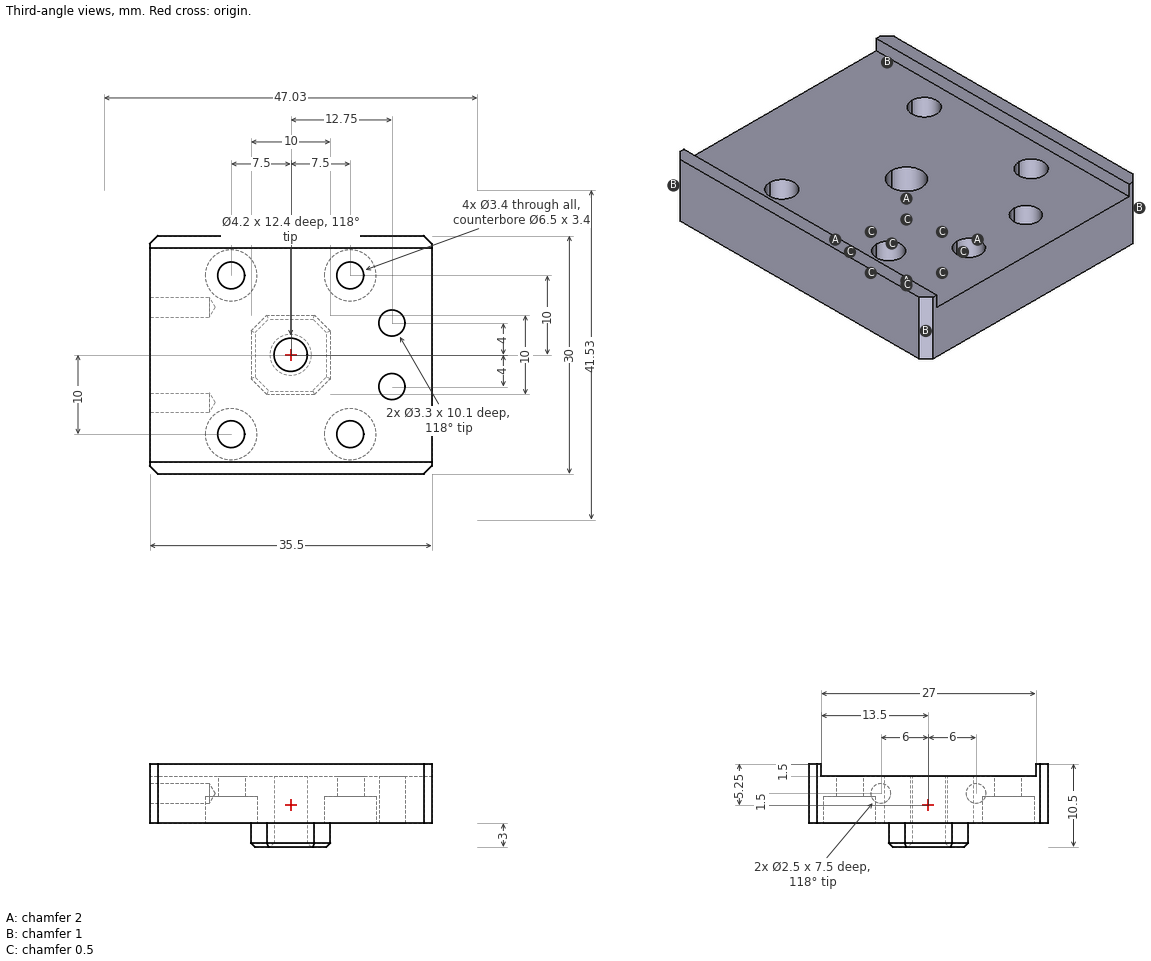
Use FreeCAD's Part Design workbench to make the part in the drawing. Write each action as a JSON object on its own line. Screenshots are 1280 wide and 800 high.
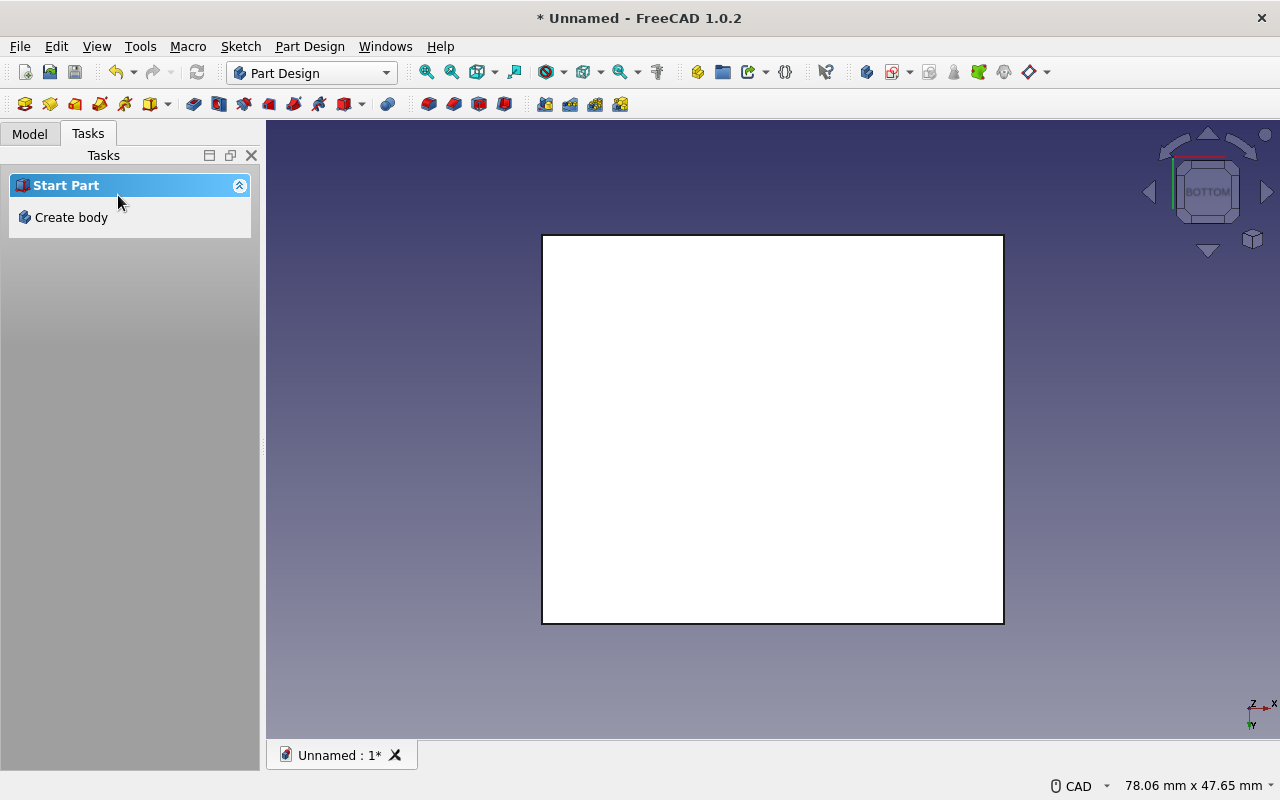
{"action": "left_click", "coordinate": [773, 428]}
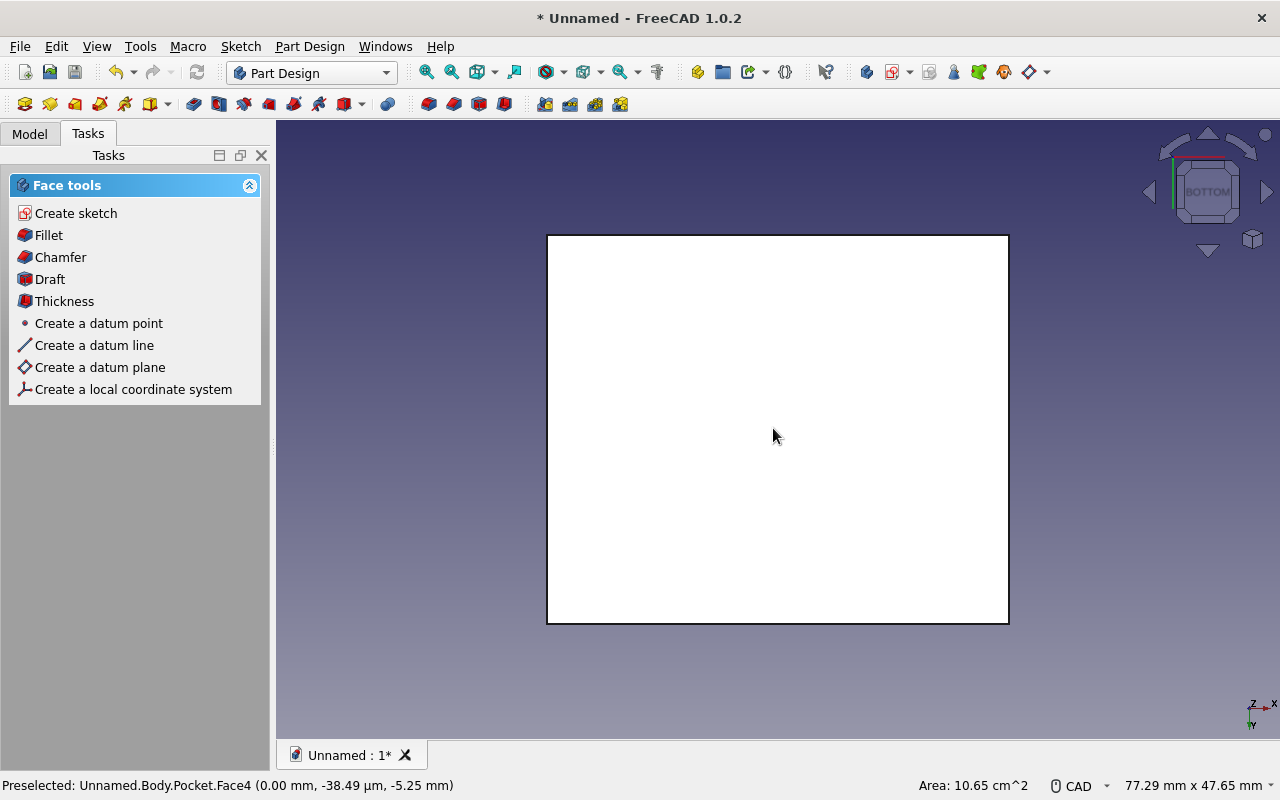
{"action": "left_click", "coordinate": [892, 72]}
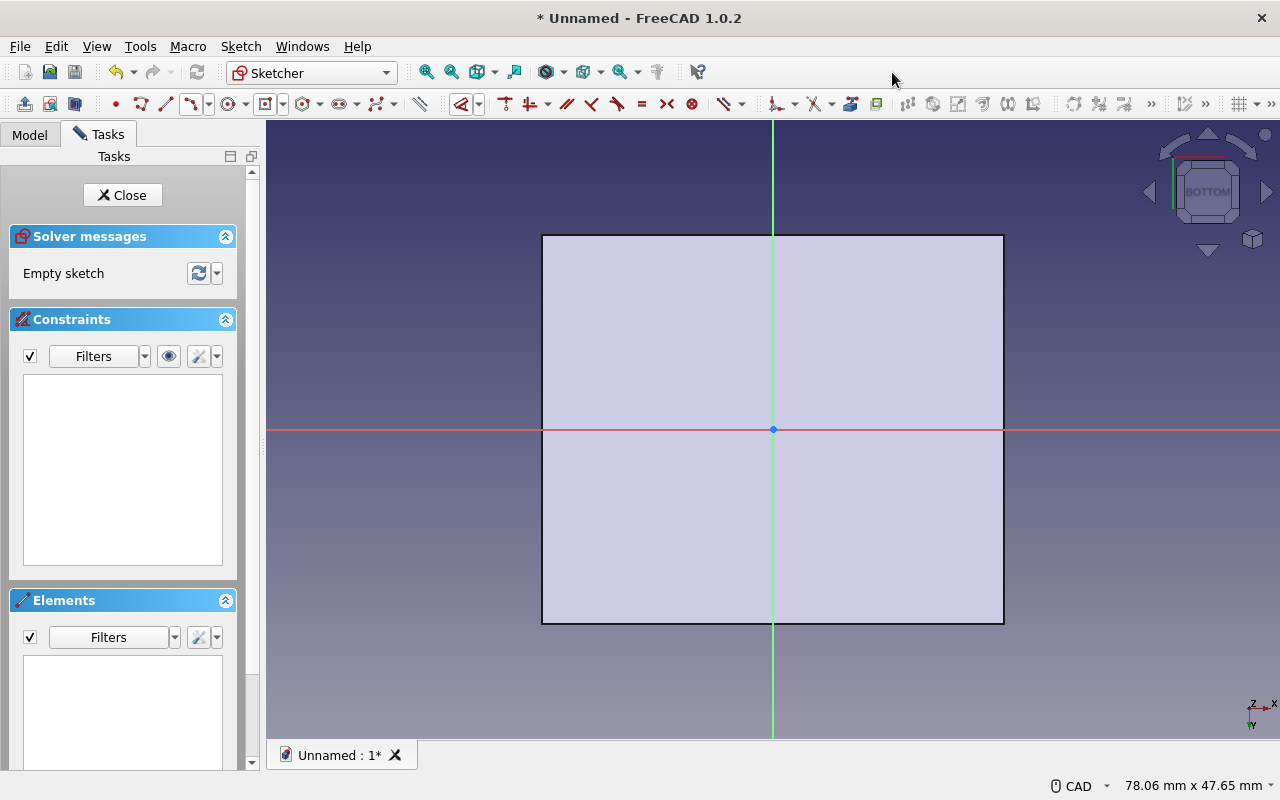
{"action": "scroll", "coordinate": [784, 430], "scroll_direction": "up", "scroll_amount": 10}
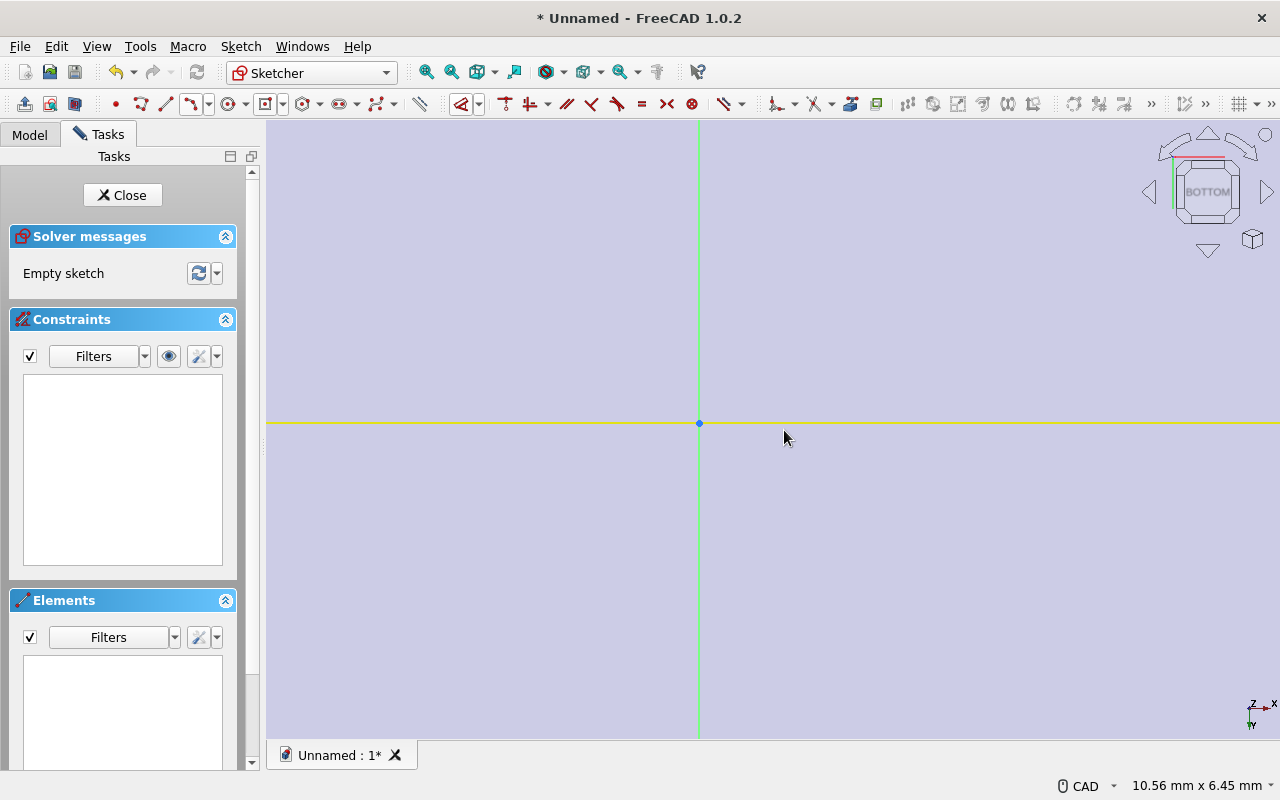
{"action": "key", "text": "g c"}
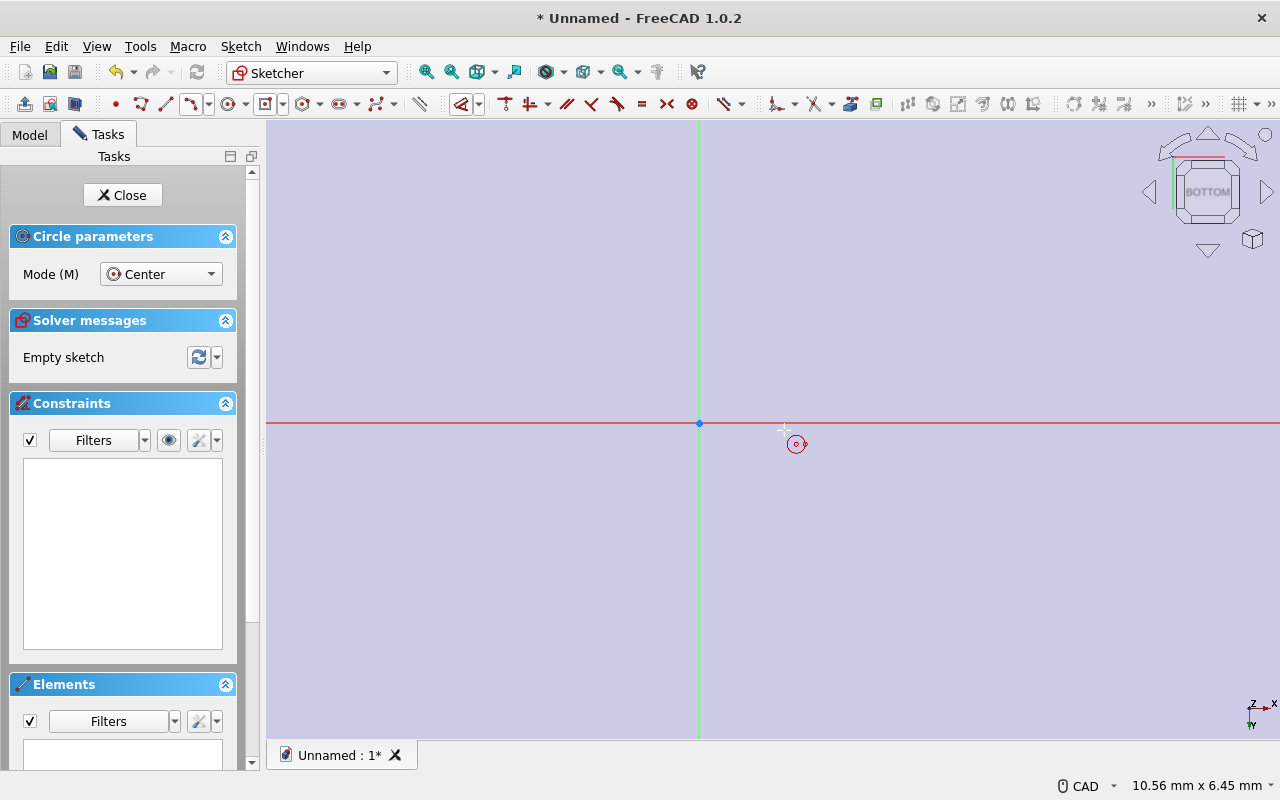
{"action": "left_click", "coordinate": [699, 423]}
{"action": "left_click", "coordinate": [842, 281]}
{"action": "key", "text": "Escape"}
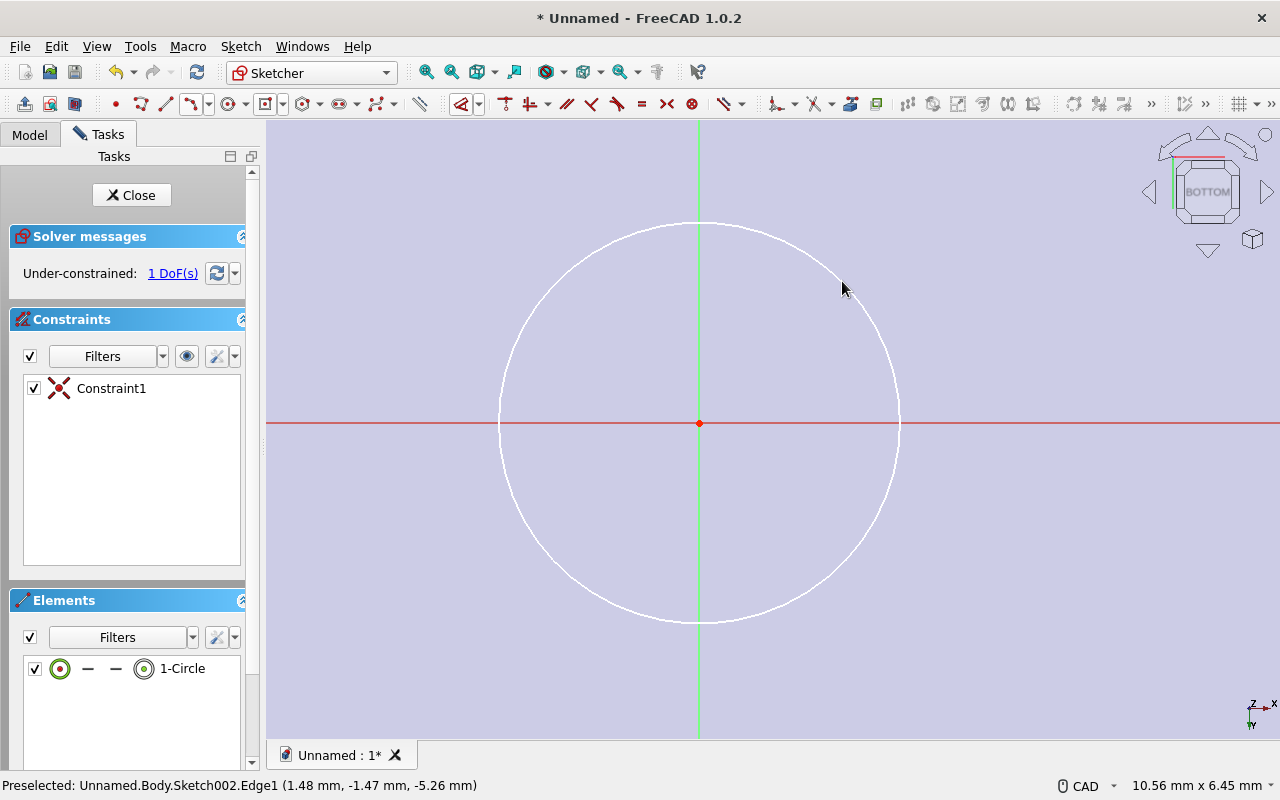
{"action": "key", "text": "d"}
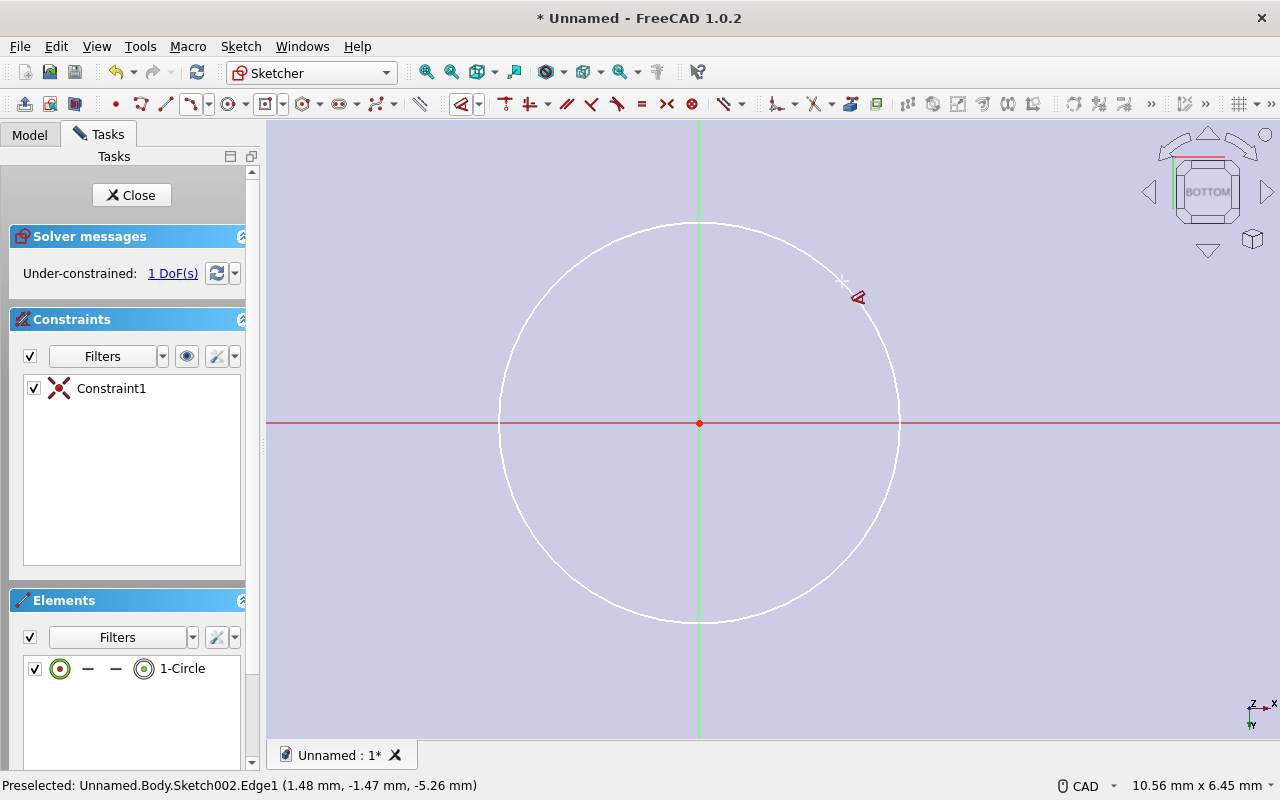
{"action": "left_click", "coordinate": [841, 281]}
{"action": "left_click", "coordinate": [864, 258]}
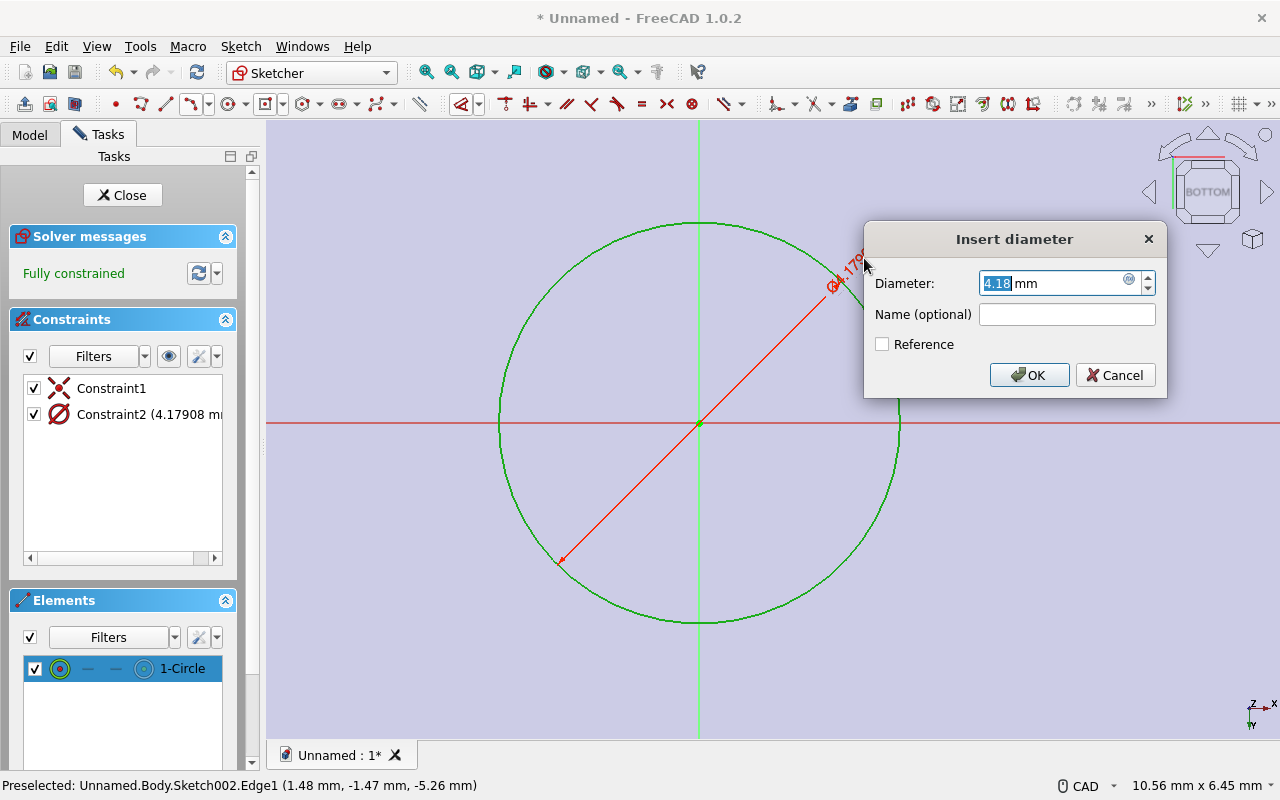
{"action": "type", "text": "4.2"}
{"action": "key", "text": "Return"}
{"action": "key", "text": "Escape"}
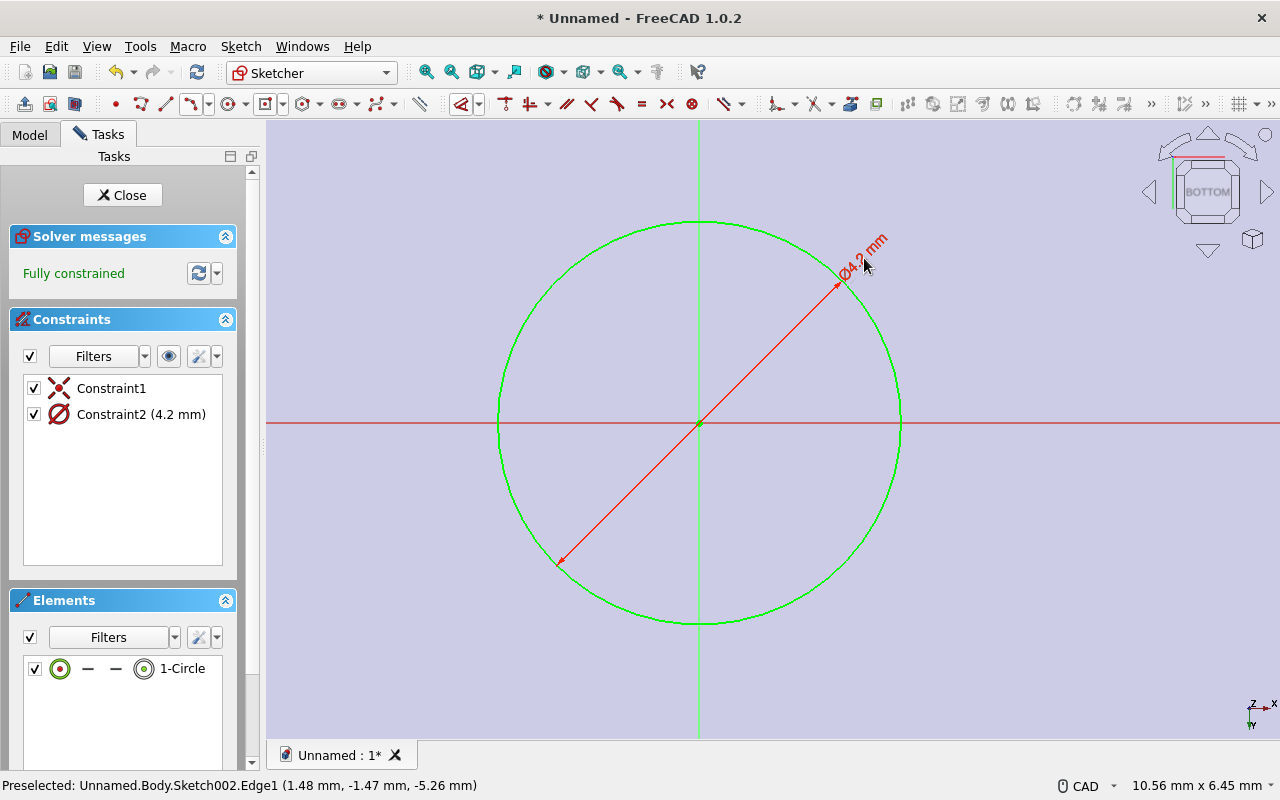
{"action": "left_click", "coordinate": [123, 195]}